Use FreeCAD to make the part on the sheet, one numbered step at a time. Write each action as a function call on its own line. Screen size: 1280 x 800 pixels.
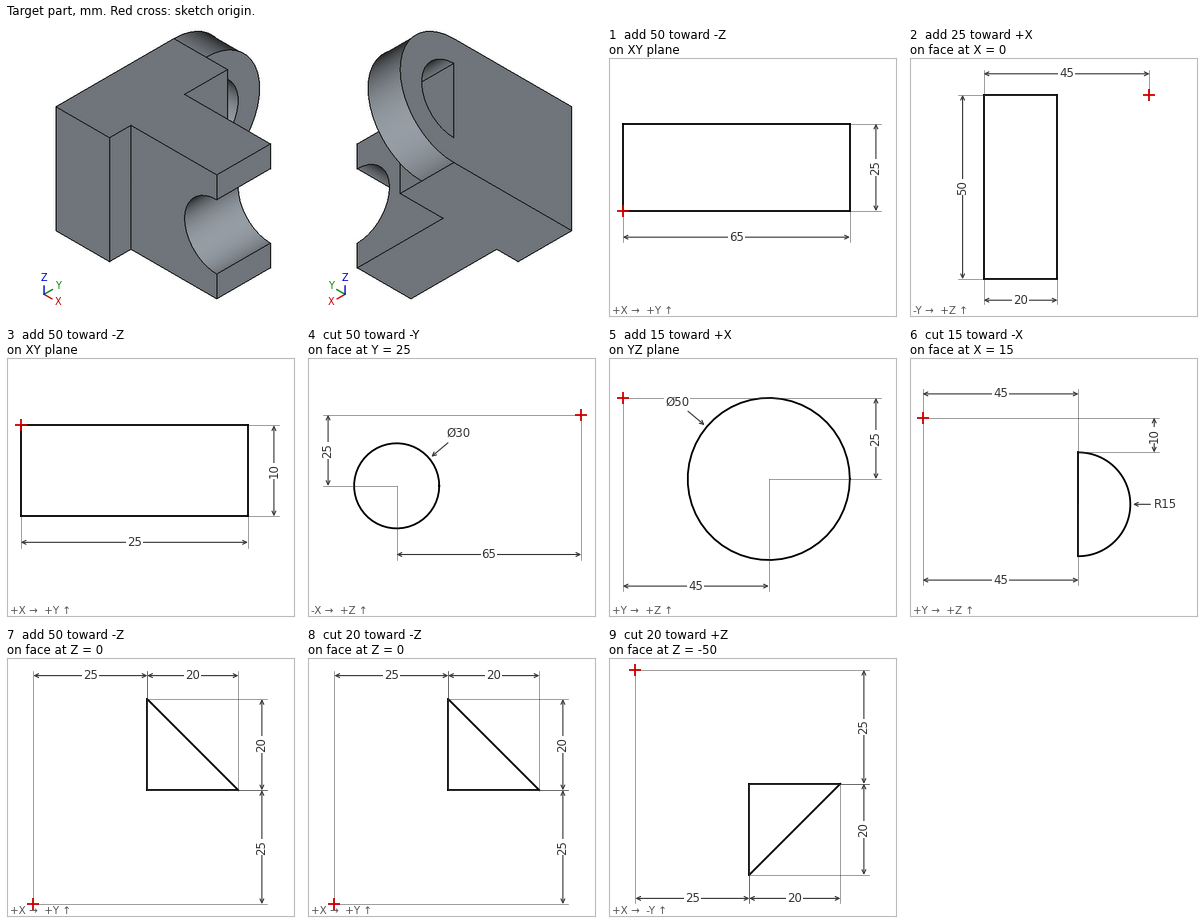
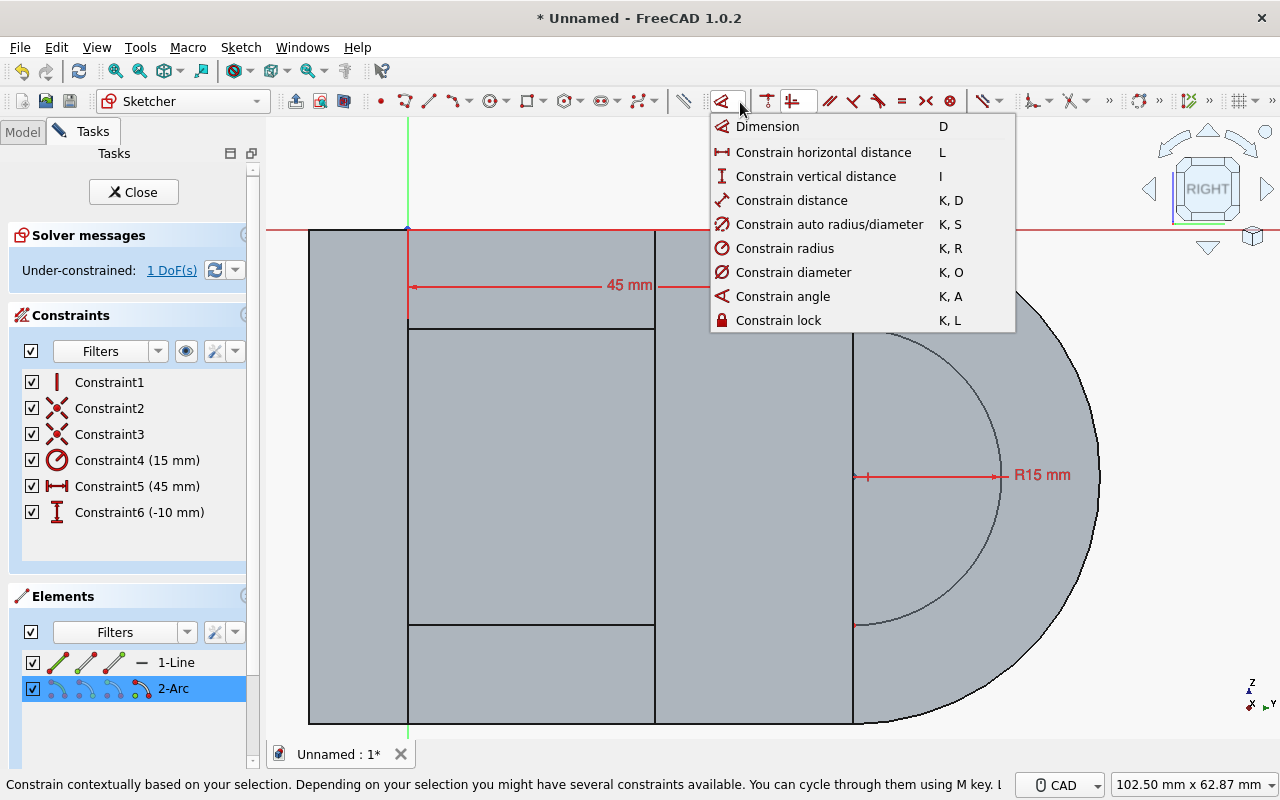
click(863, 152)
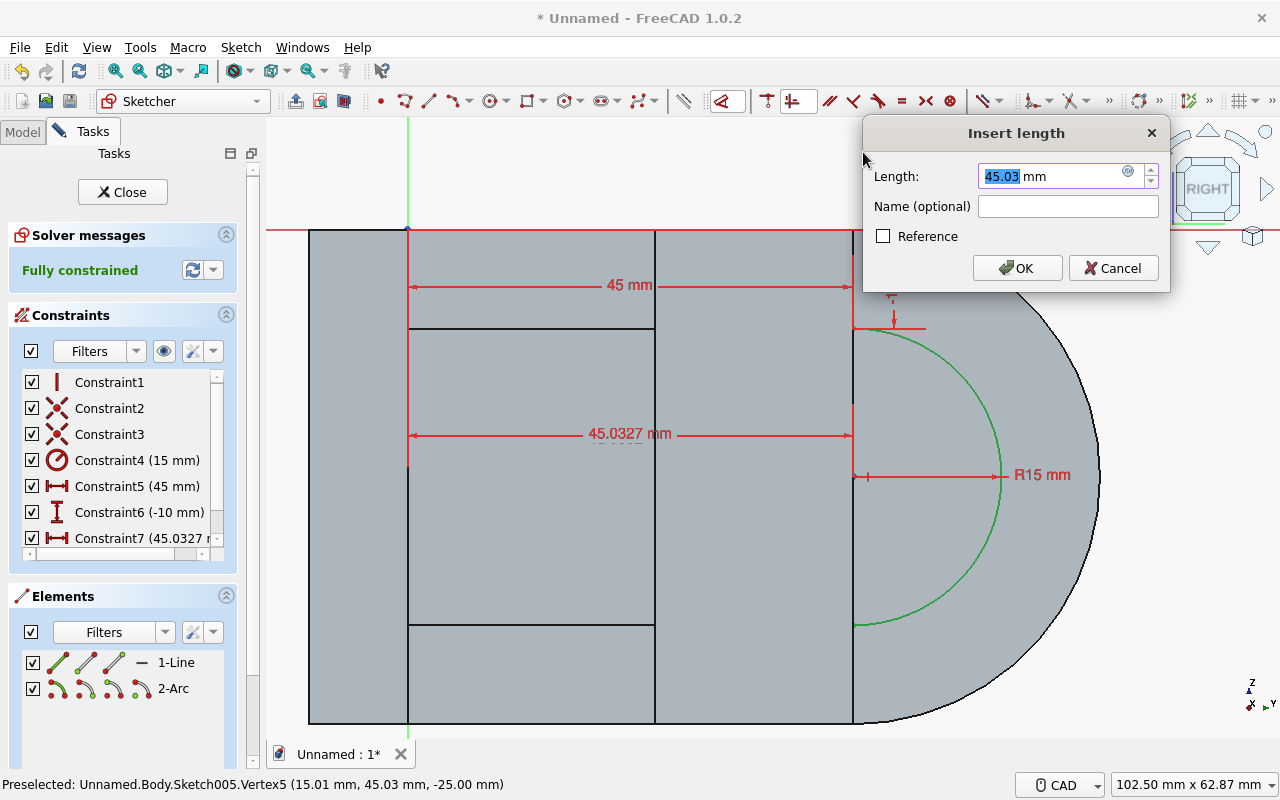
text(45)
key(Return)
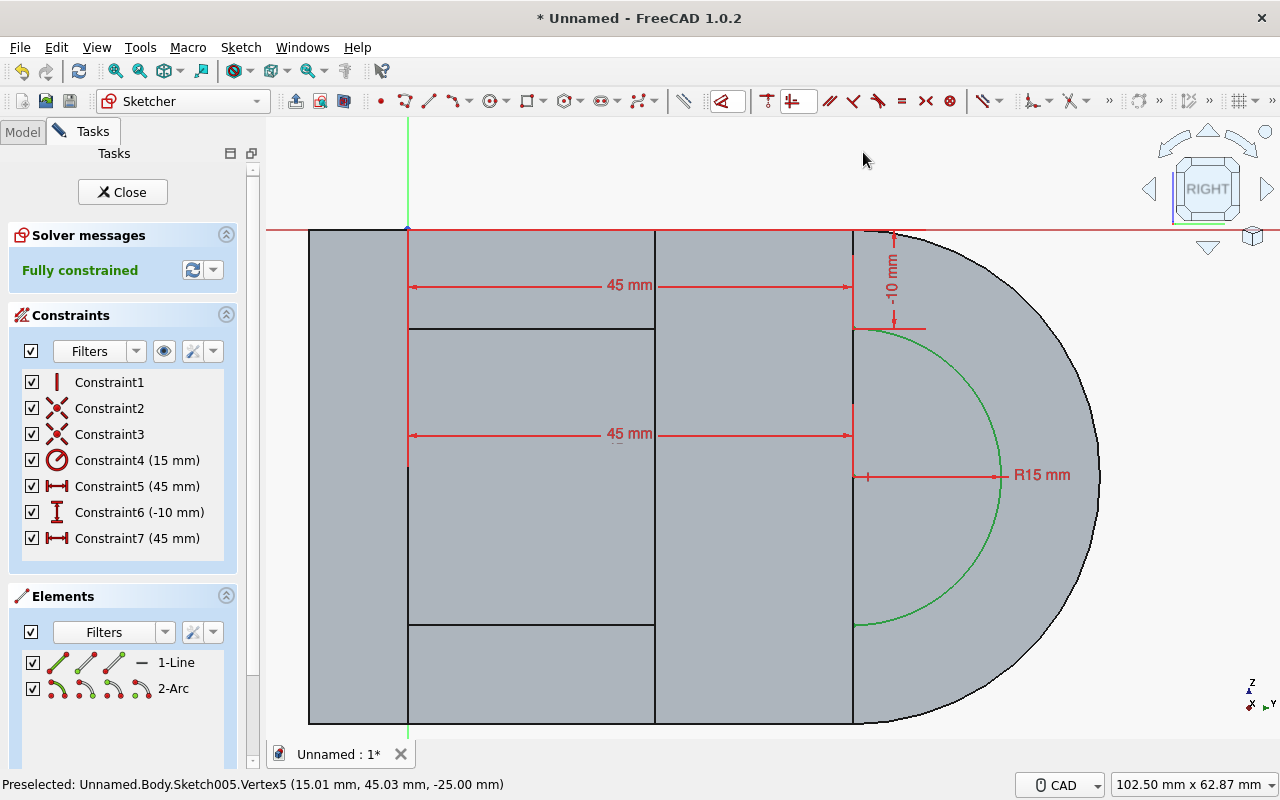
click(123, 192)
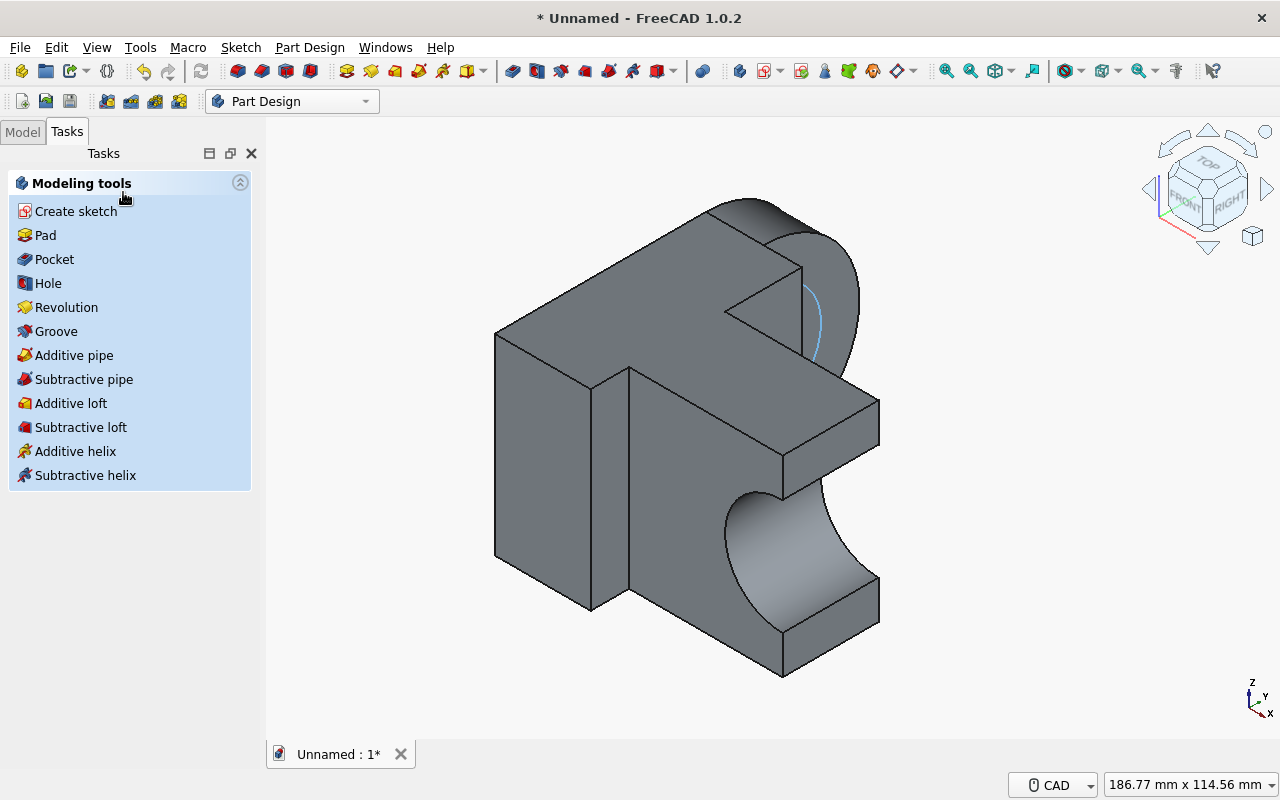
click(514, 72)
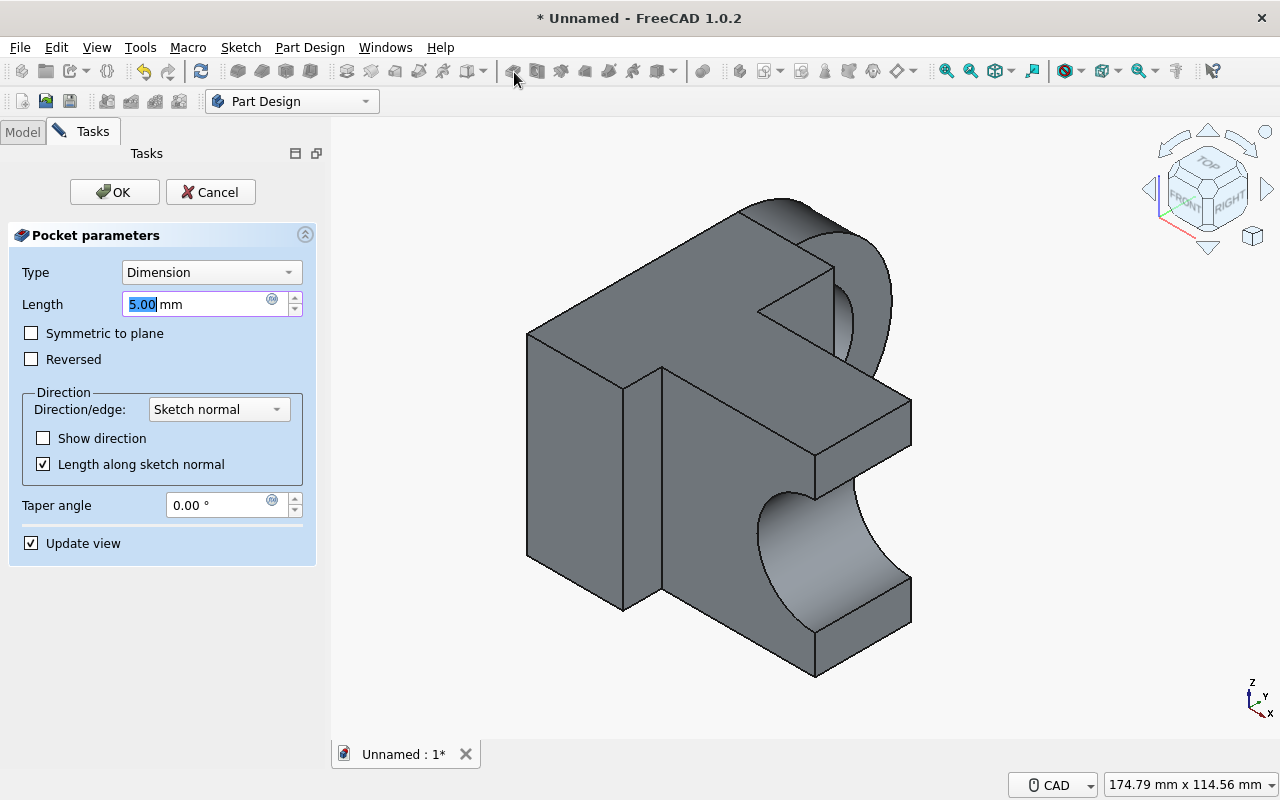
text(15)
key(Tab)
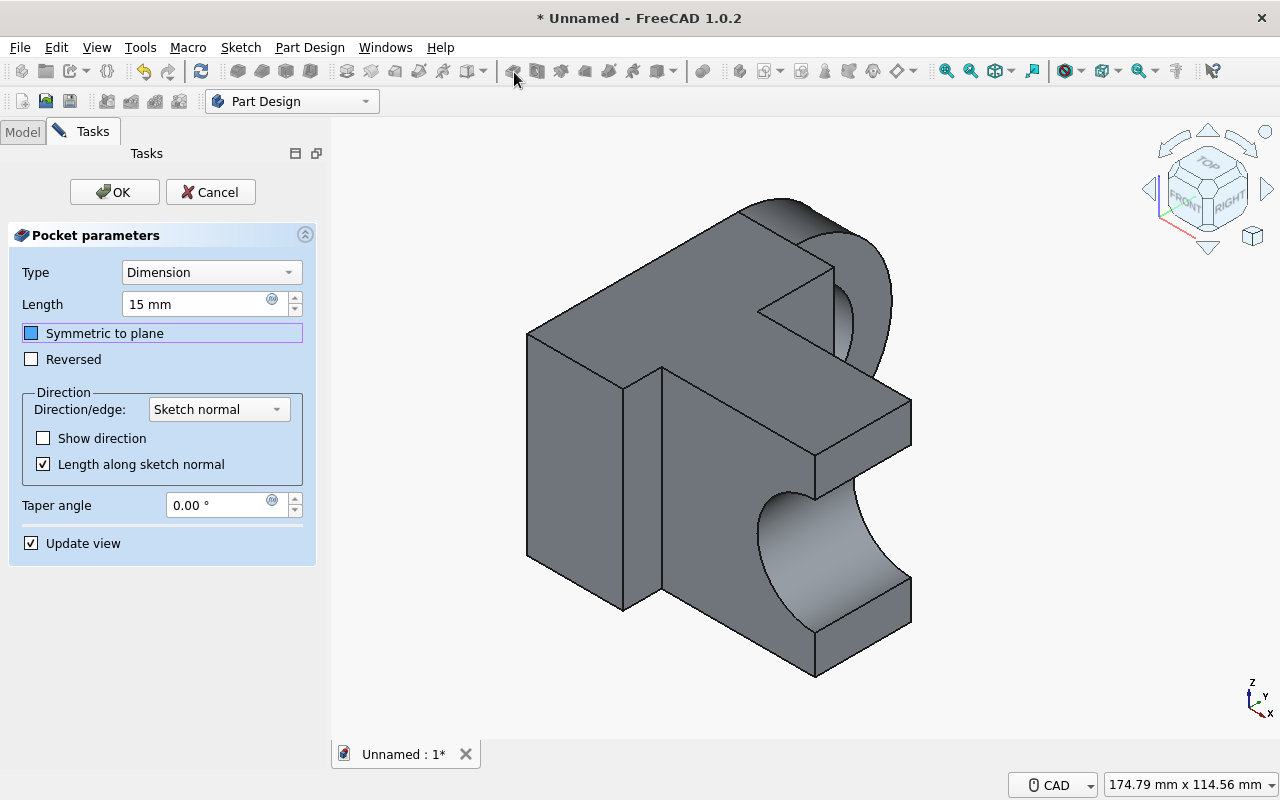
click(115, 192)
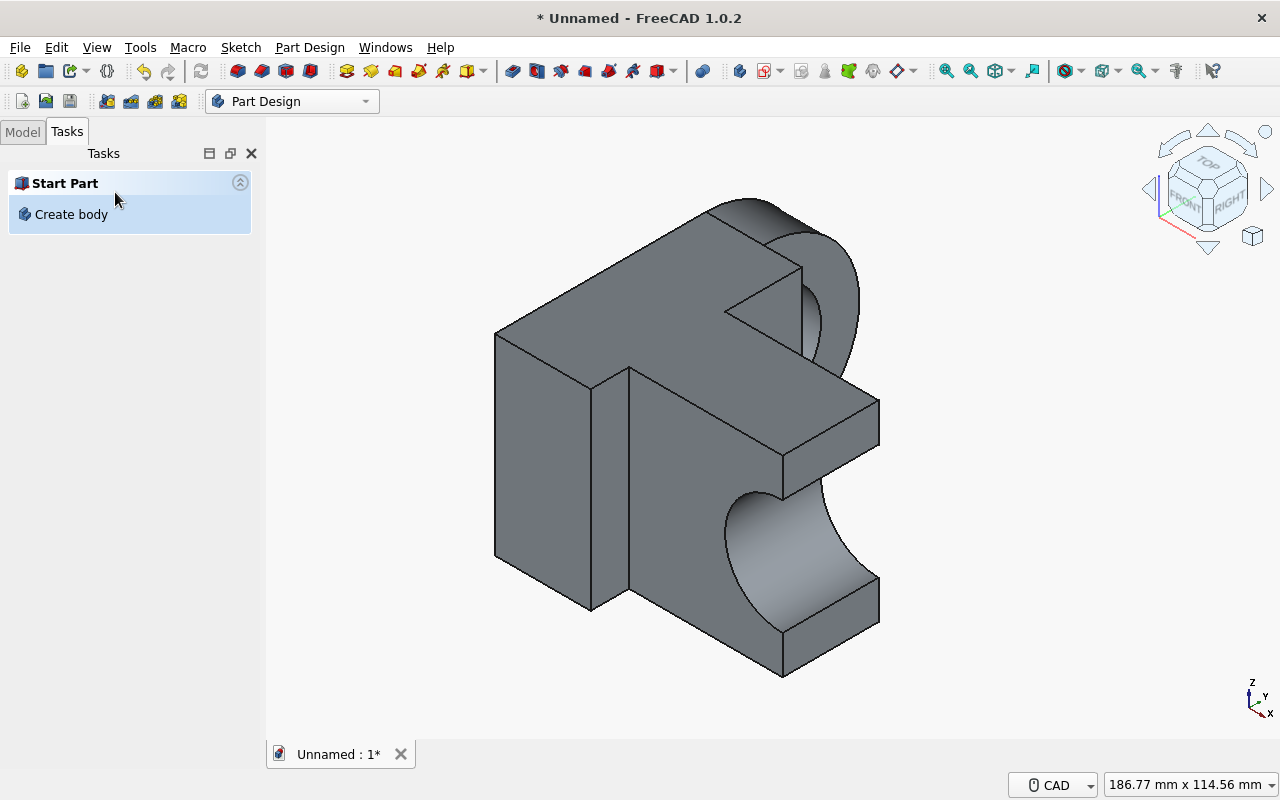
click(624, 320)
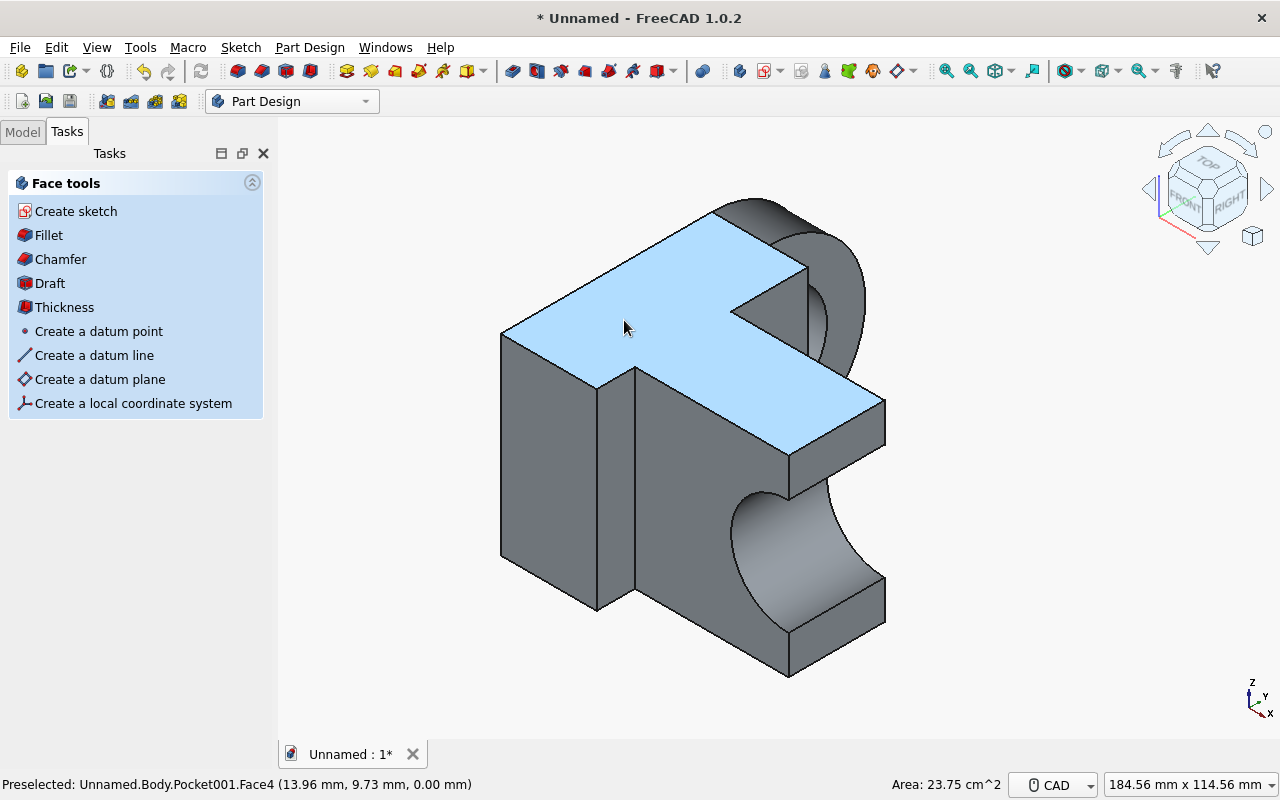
click(764, 72)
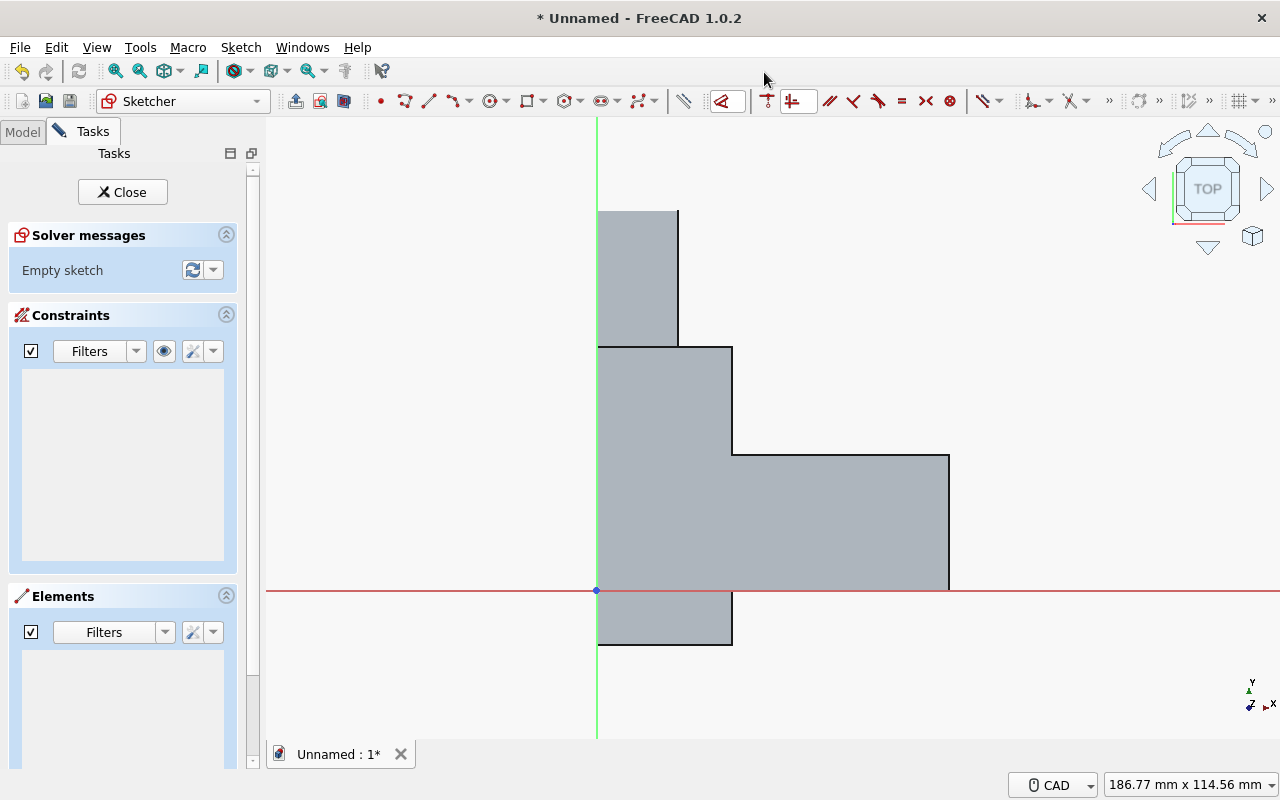
scroll(748, 552, up, 2)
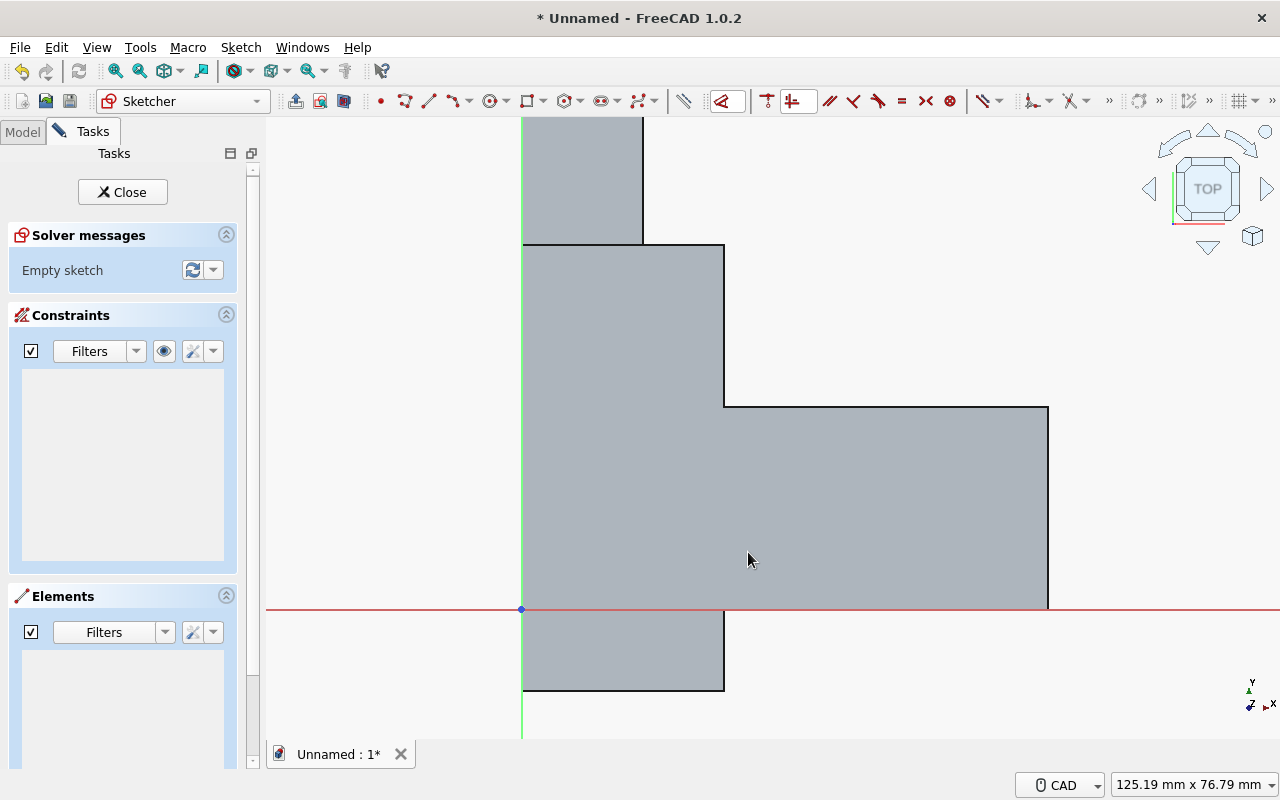
click(406, 102)